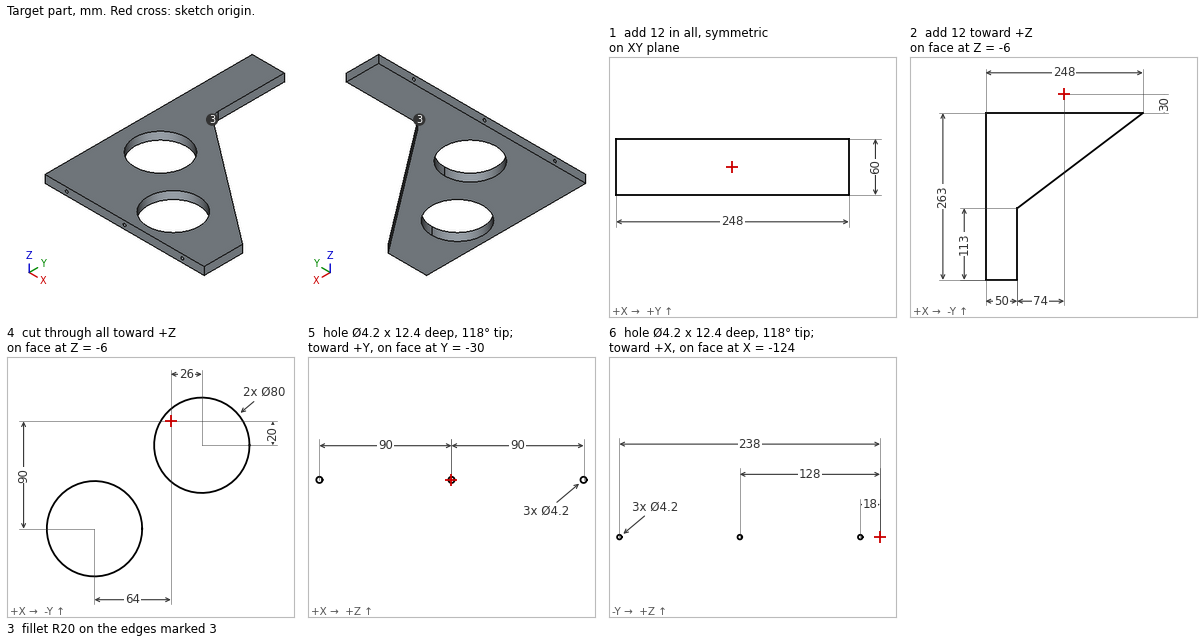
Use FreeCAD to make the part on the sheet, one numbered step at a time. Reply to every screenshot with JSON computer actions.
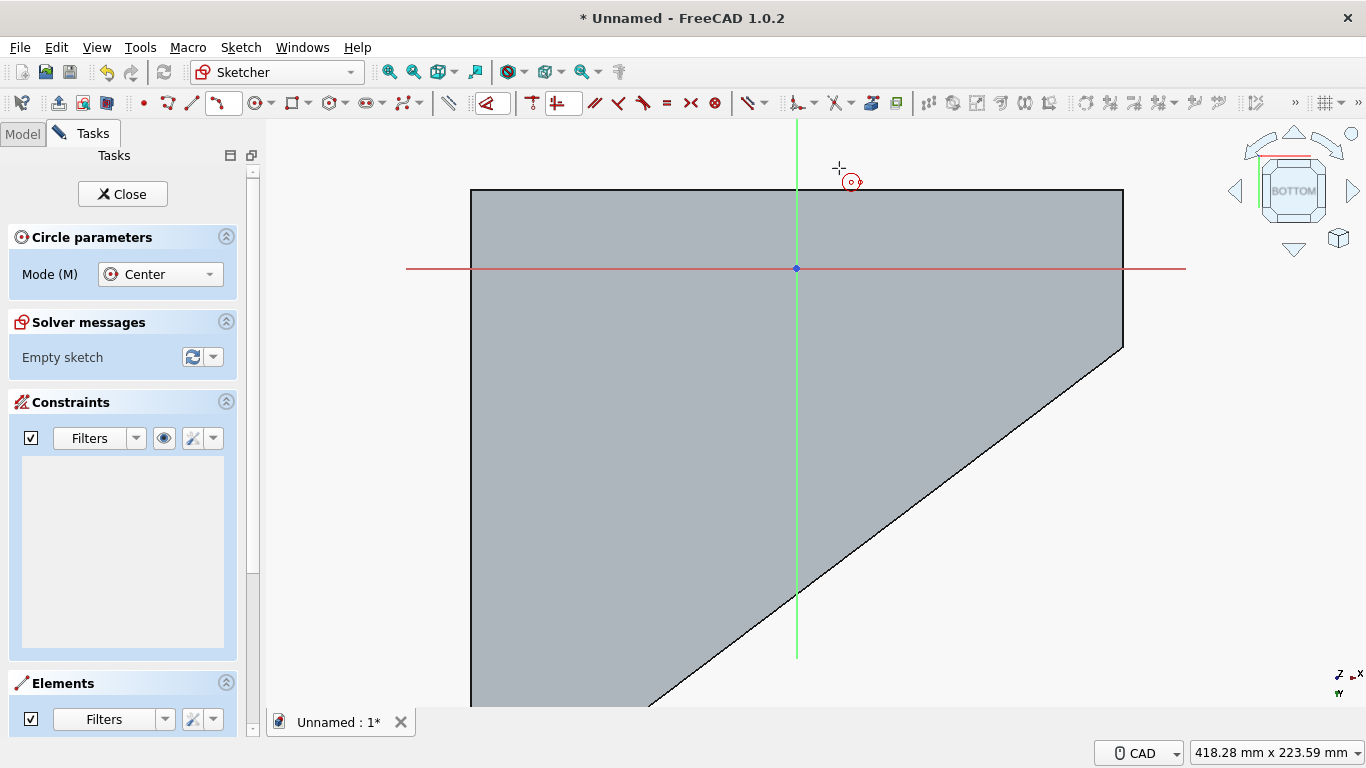
{"action": "left_click", "coordinate": [865, 321]}
{"action": "mouse_move", "coordinate": [939, 247]}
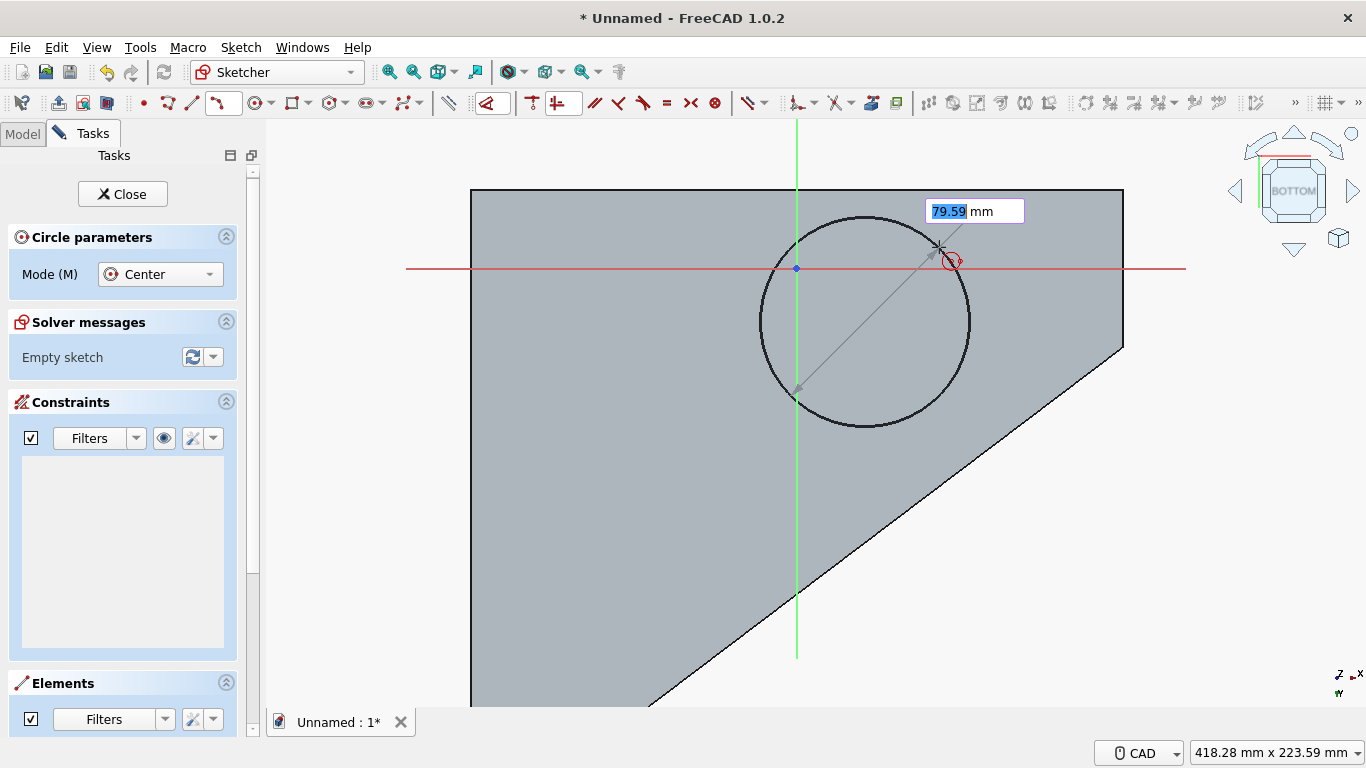
{"action": "type", "text": "80"}
{"action": "key", "text": "Return"}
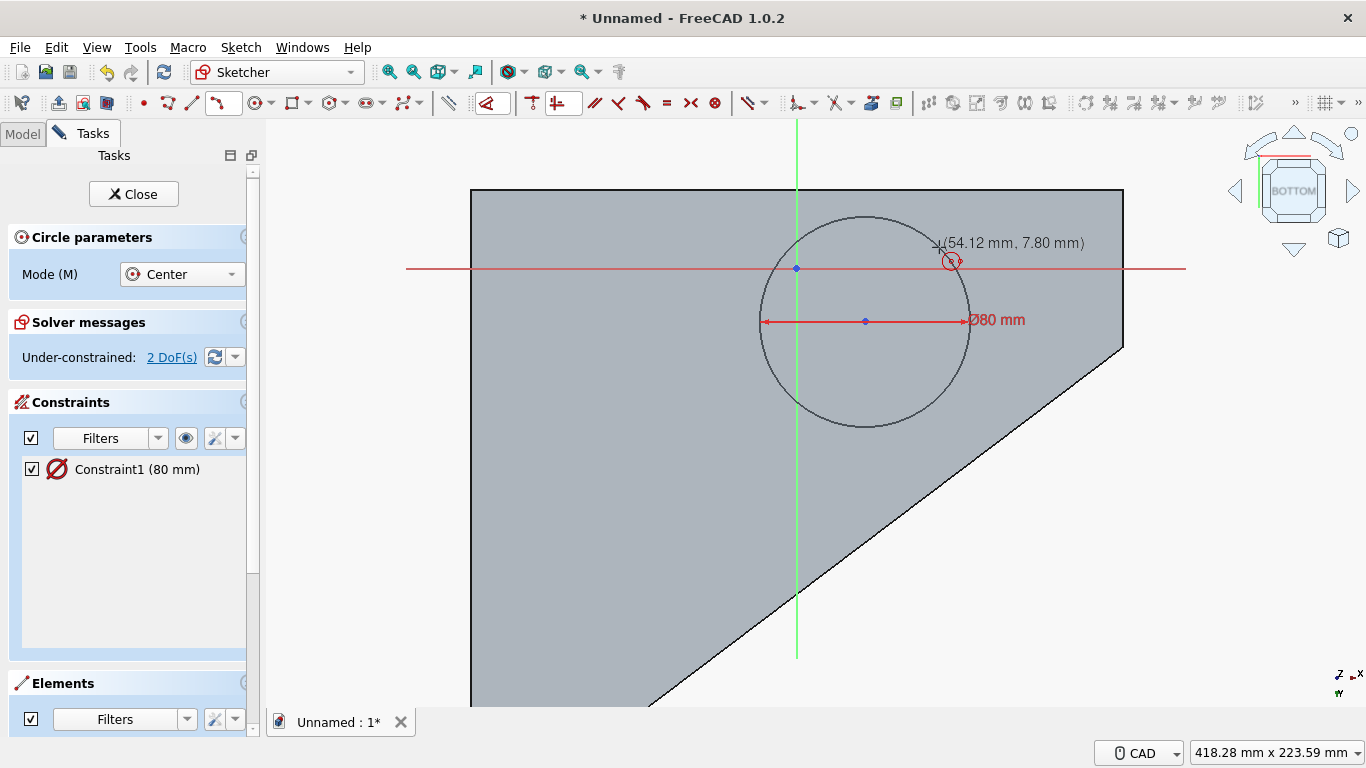
{"action": "left_click", "coordinate": [628, 505]}
{"action": "mouse_move", "coordinate": [703, 431]}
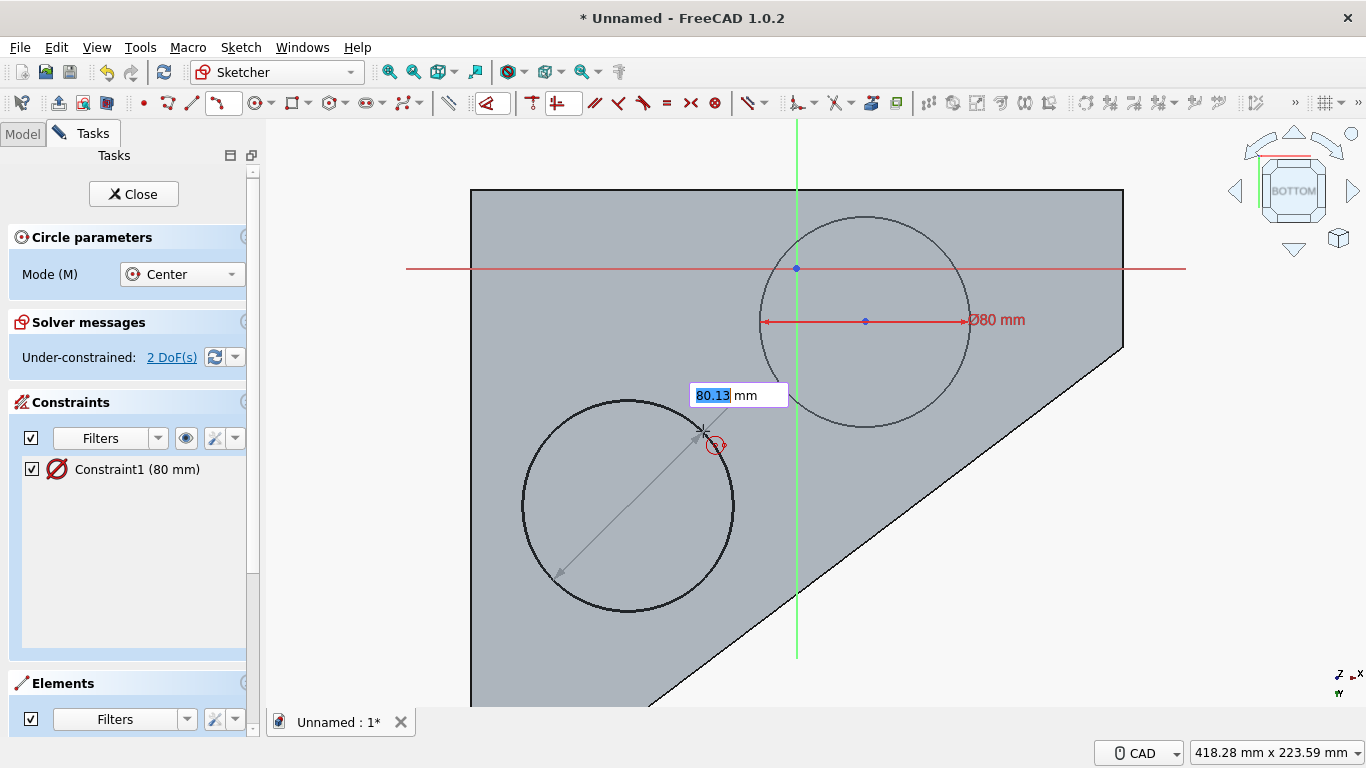
{"action": "type", "text": "80"}
{"action": "key", "text": "Return"}
{"action": "key", "text": "Escape"}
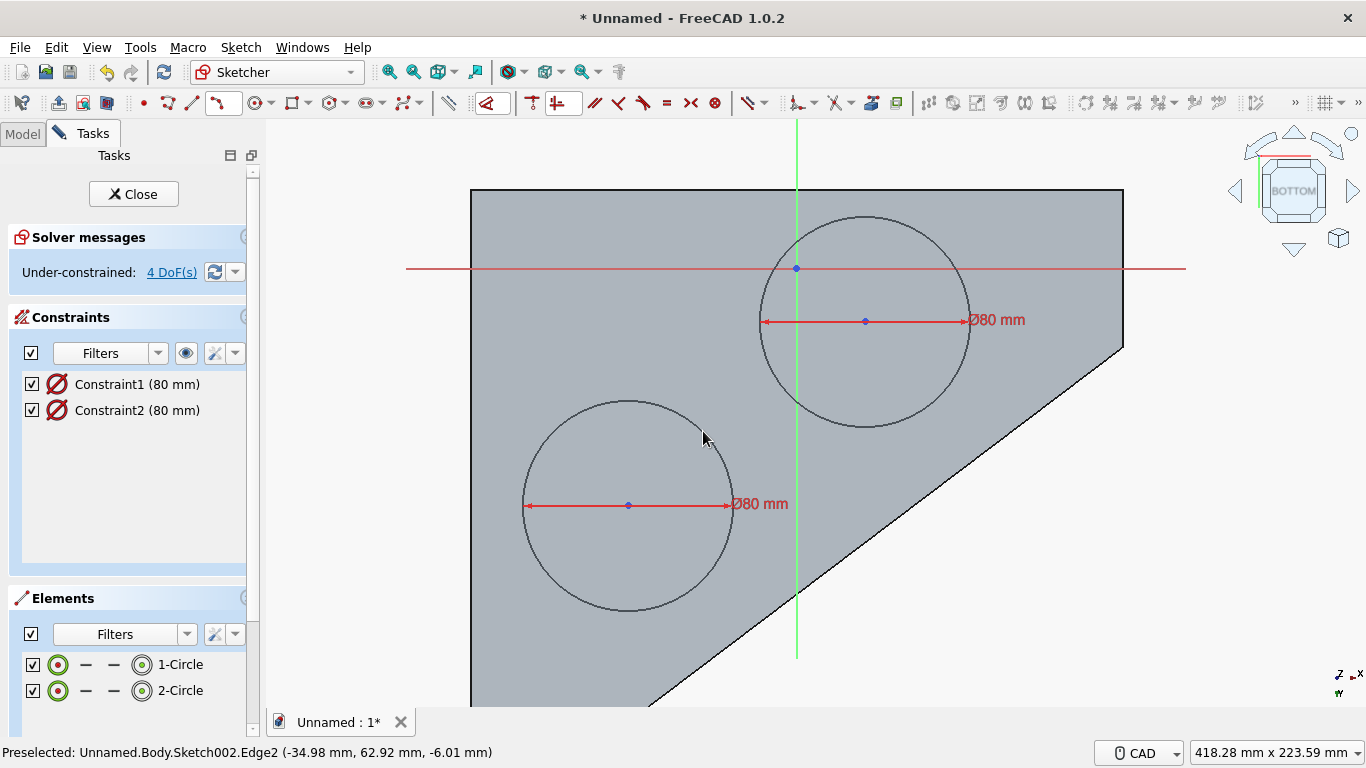
{"action": "left_click", "coordinate": [865, 322]}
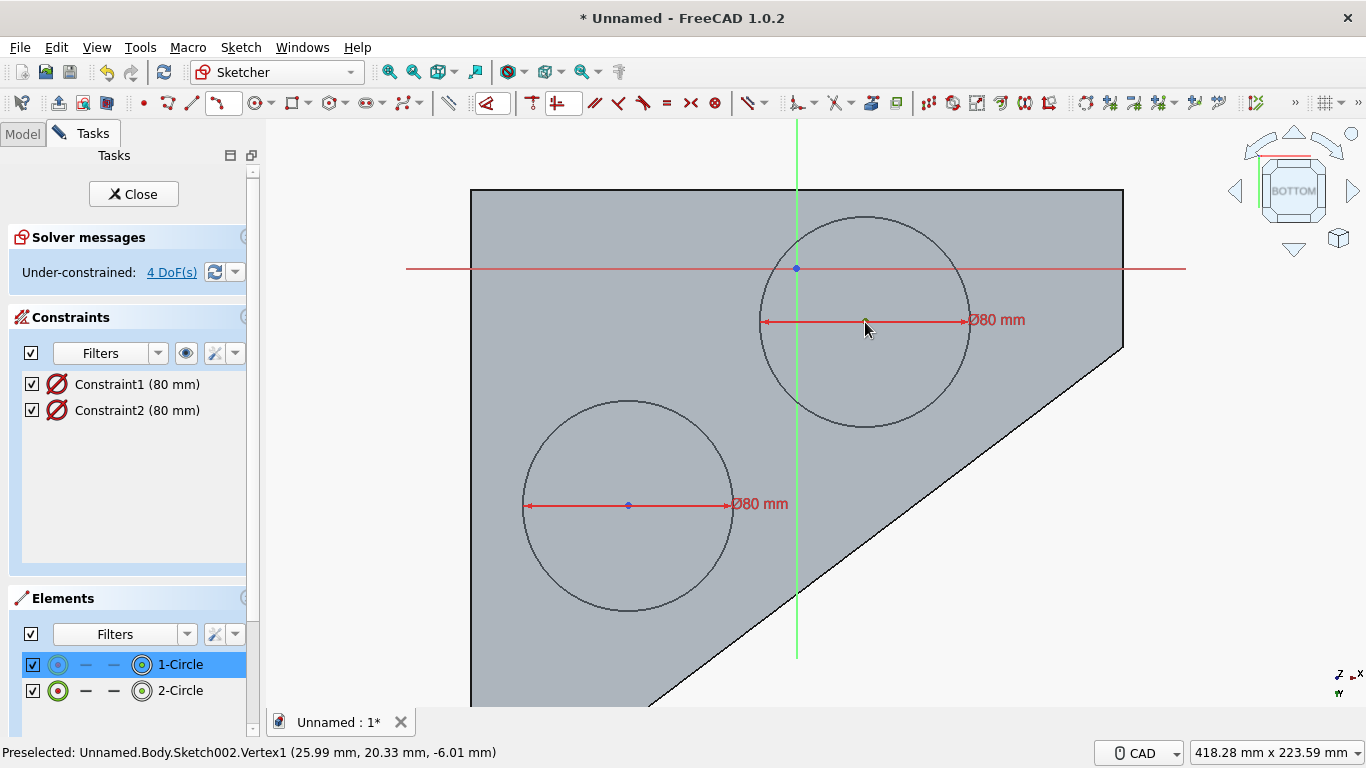
{"action": "key", "text": "l"}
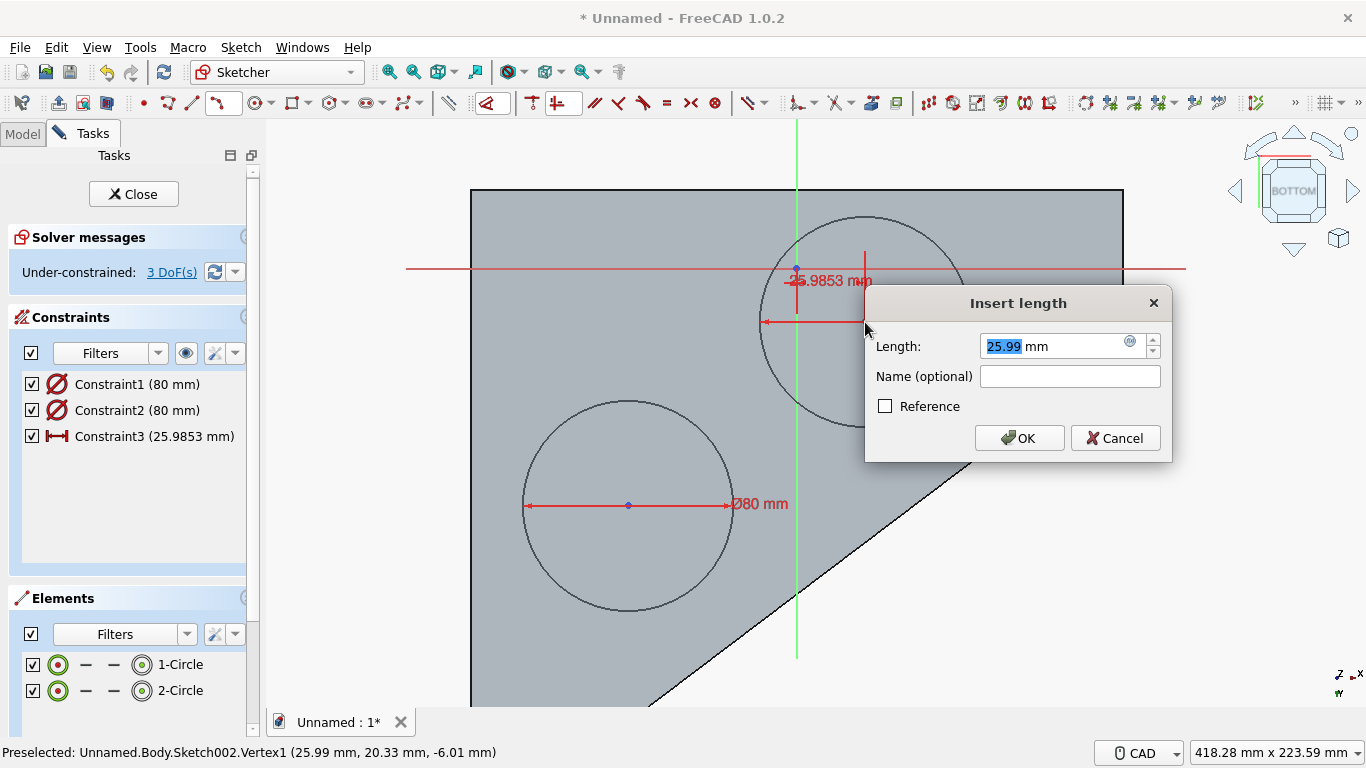
{"action": "type", "text": "26"}
{"action": "key", "text": "Return"}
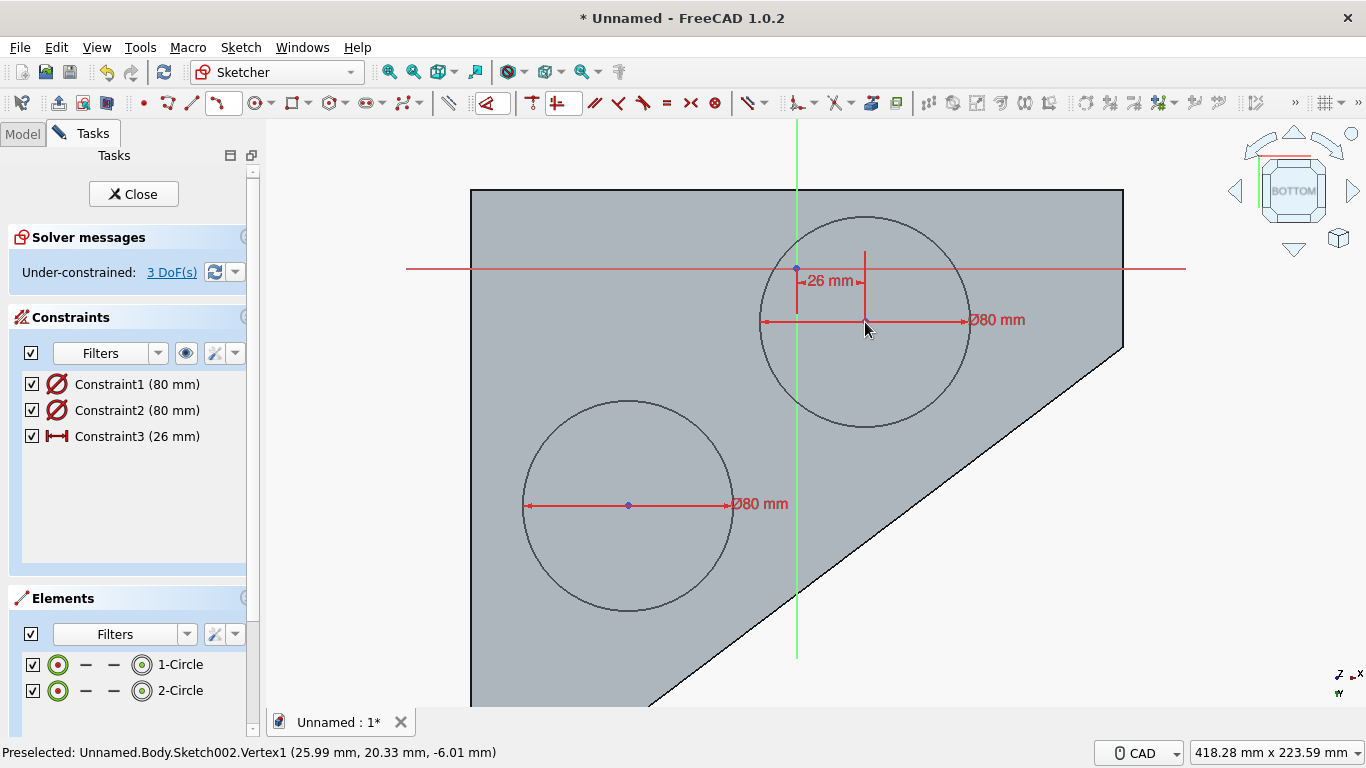
{"action": "left_click", "coordinate": [865, 322]}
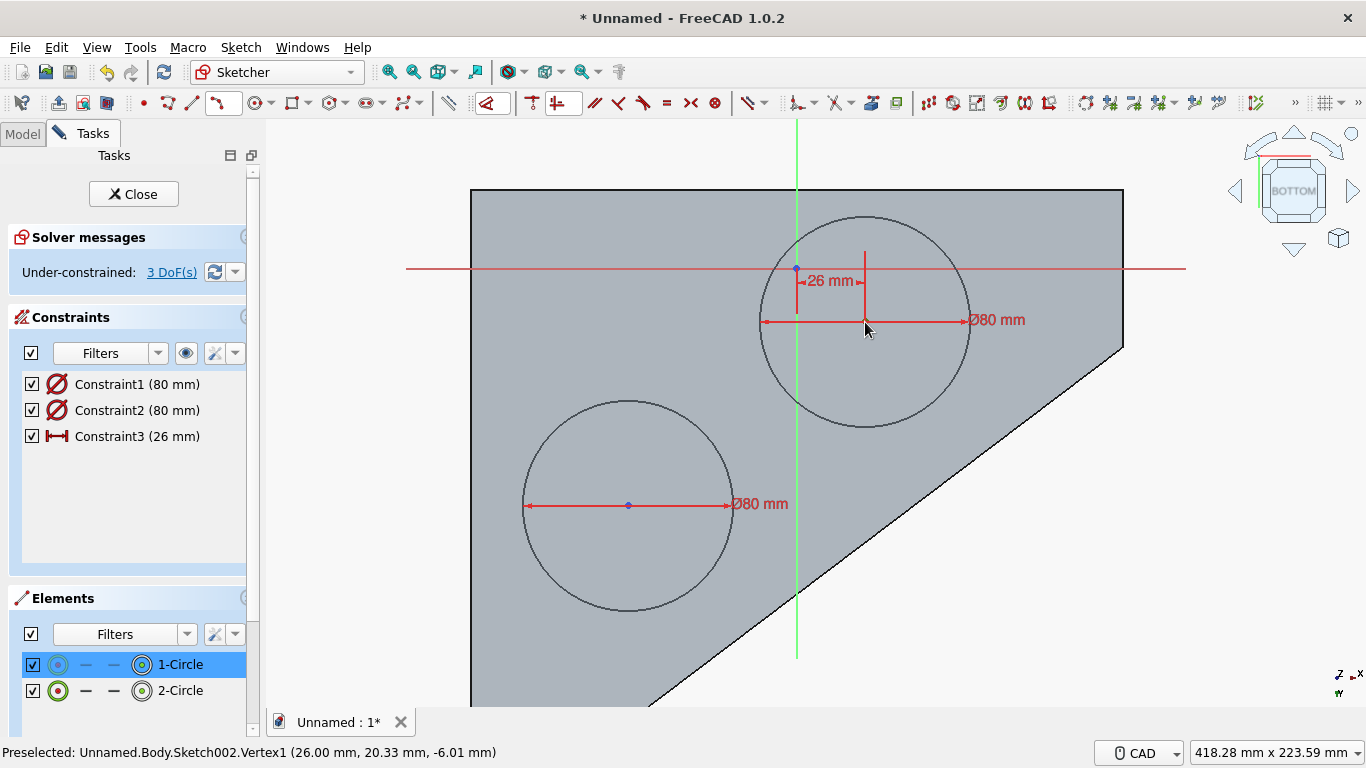
{"action": "key", "text": "i"}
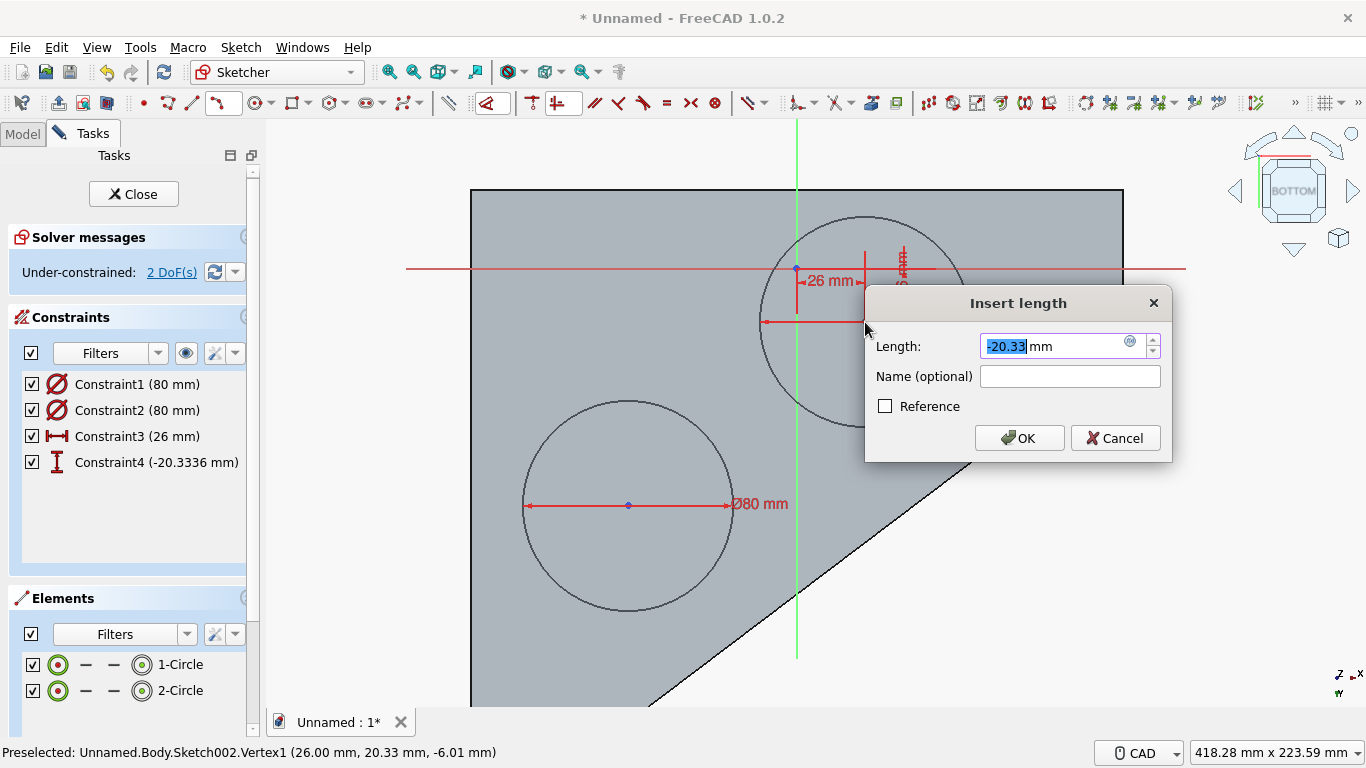
{"action": "type", "text": "-20"}
{"action": "key", "text": "Return"}